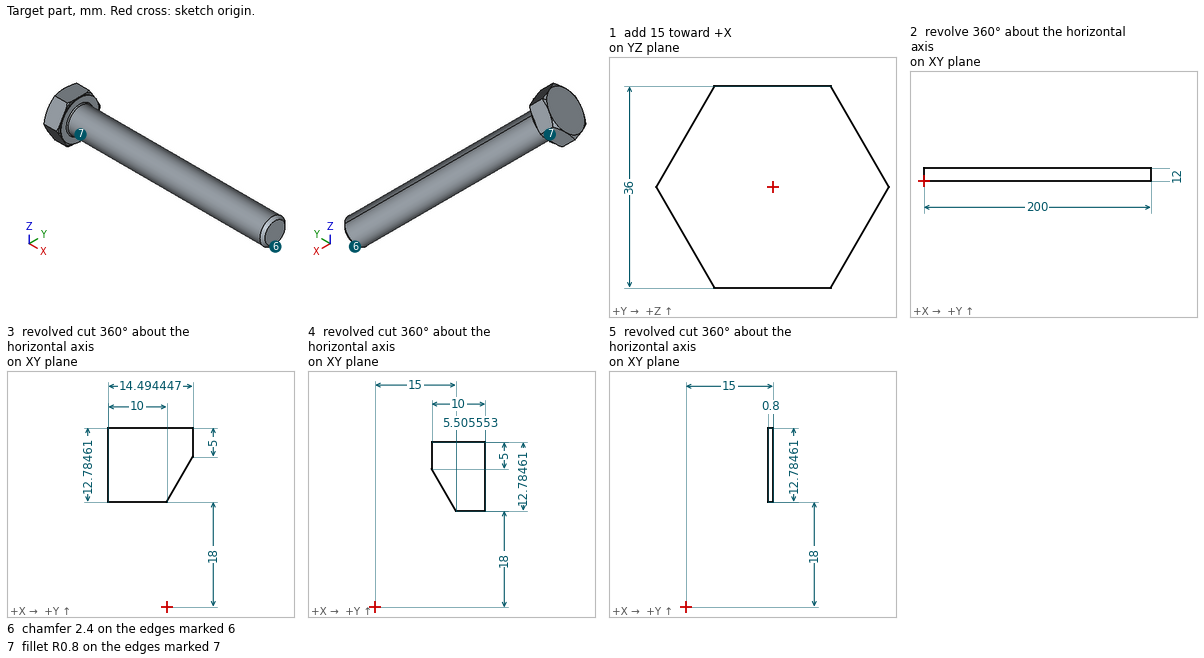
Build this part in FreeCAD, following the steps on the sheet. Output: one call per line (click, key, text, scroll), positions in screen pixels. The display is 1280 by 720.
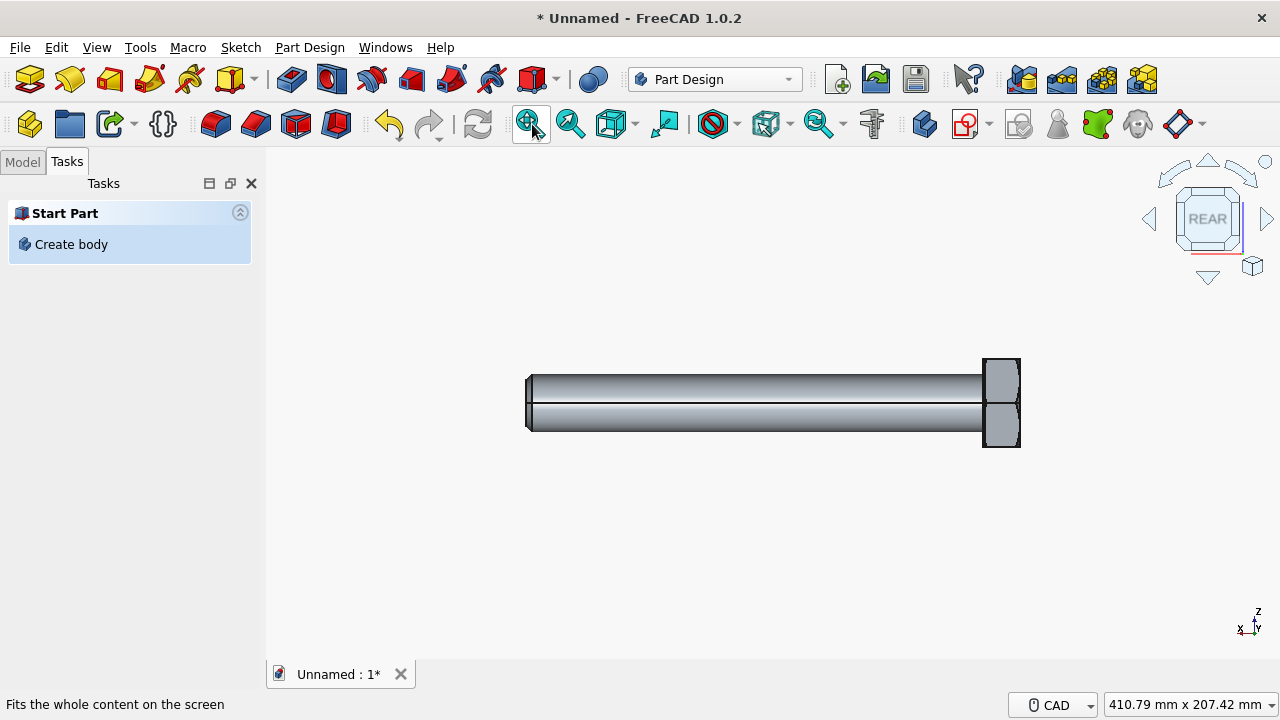
key(6)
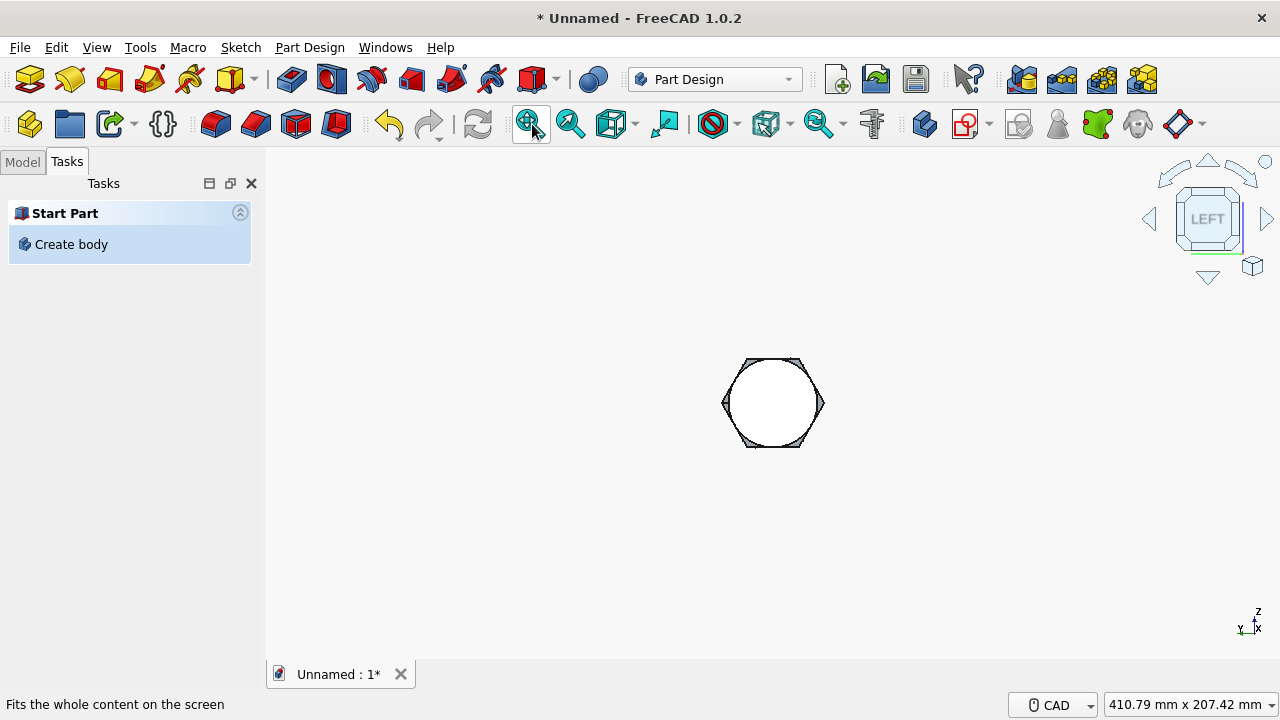
click(532, 124)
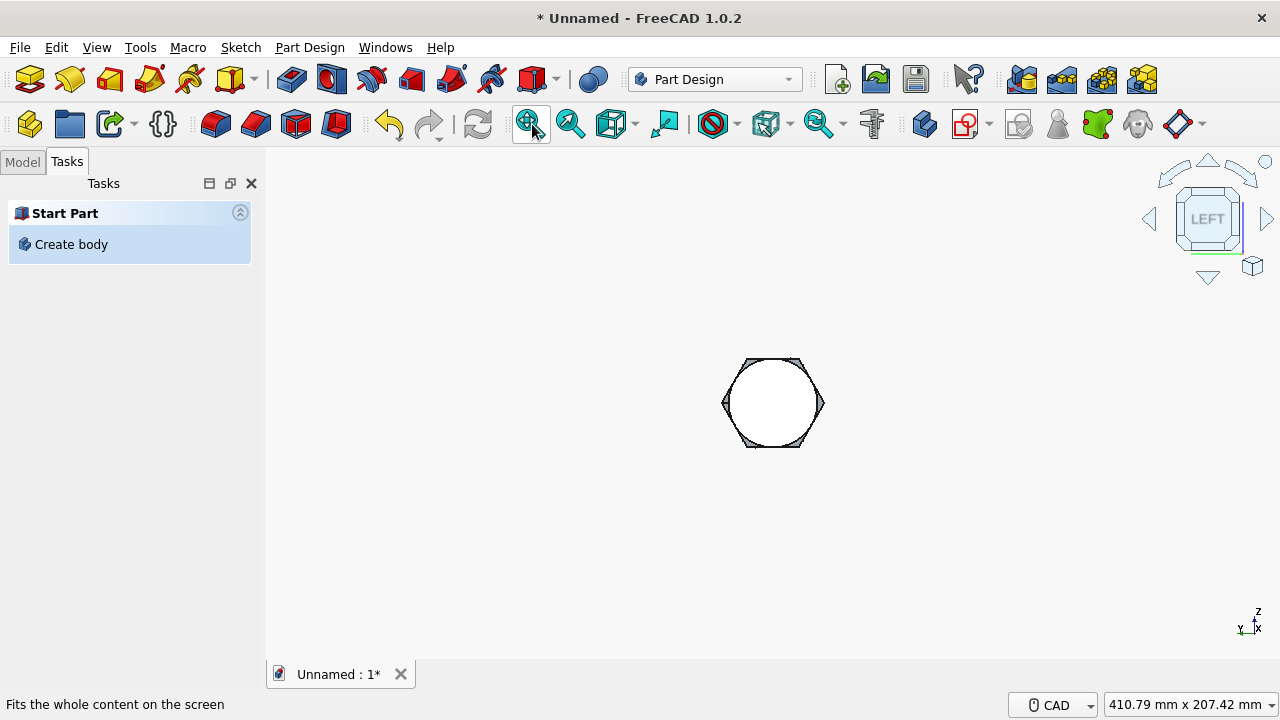
key(v)
key(3)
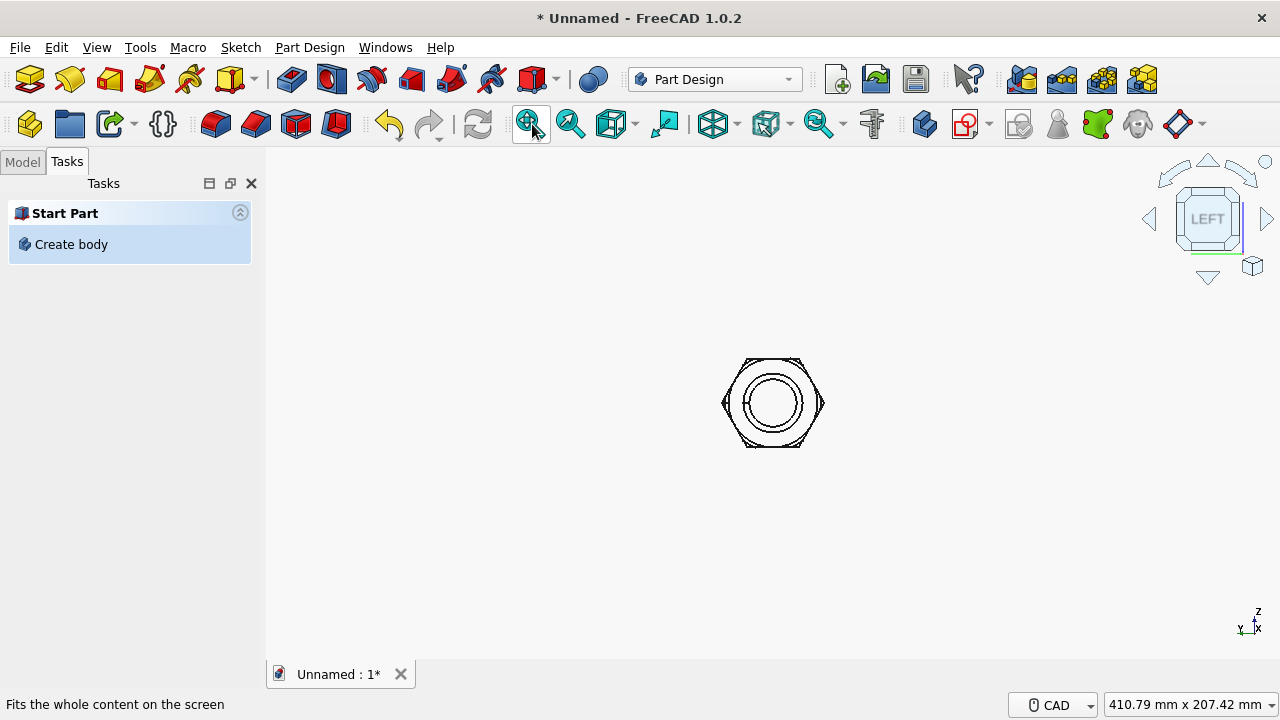
key(0)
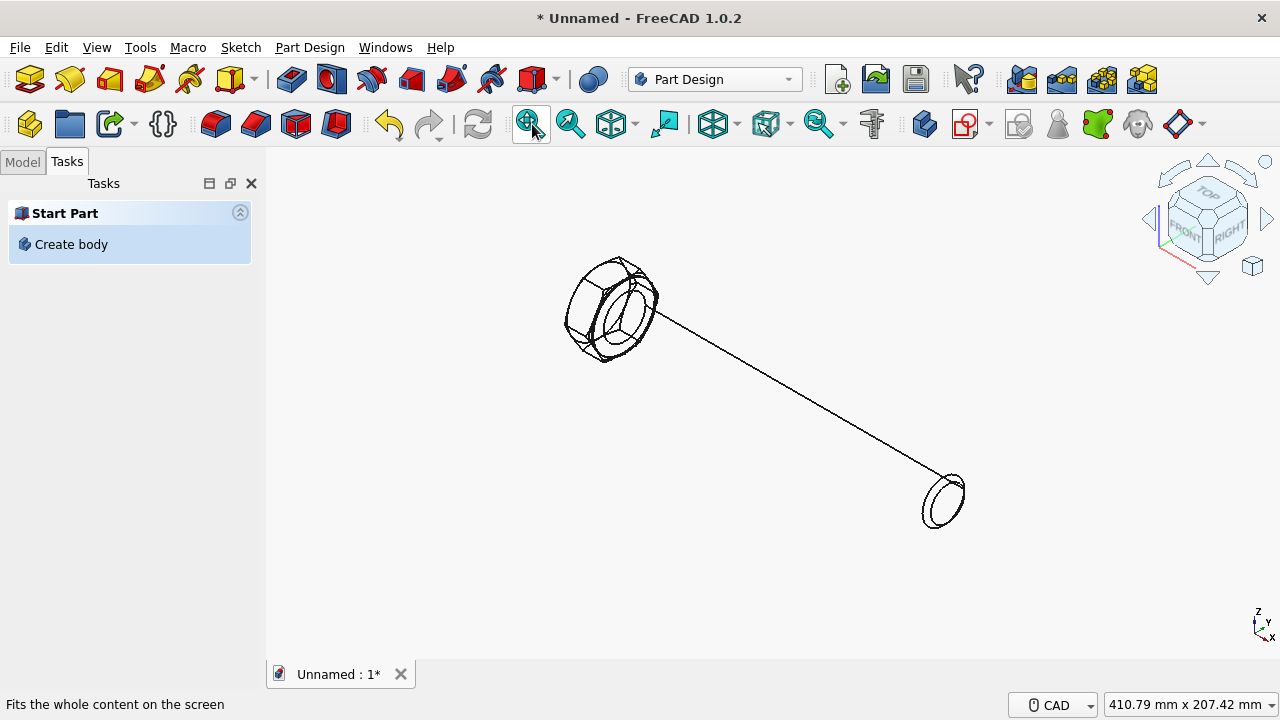
click(604, 328)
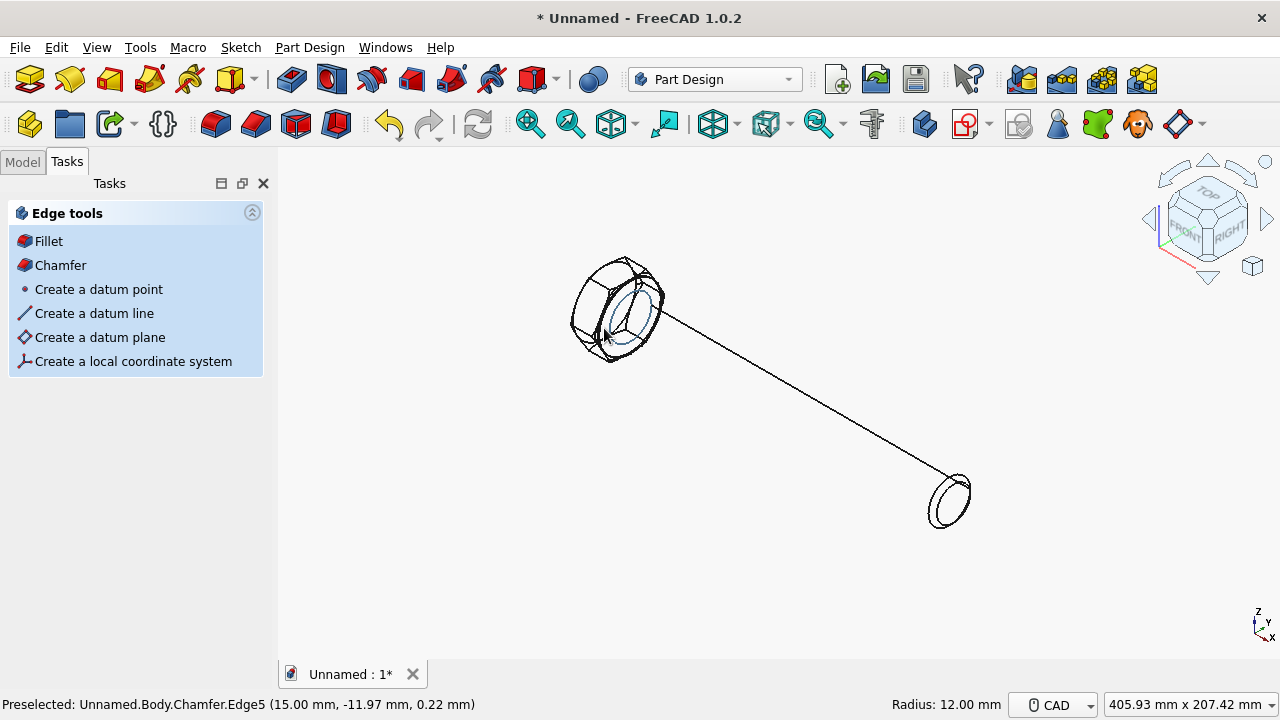
key(v)
key(1)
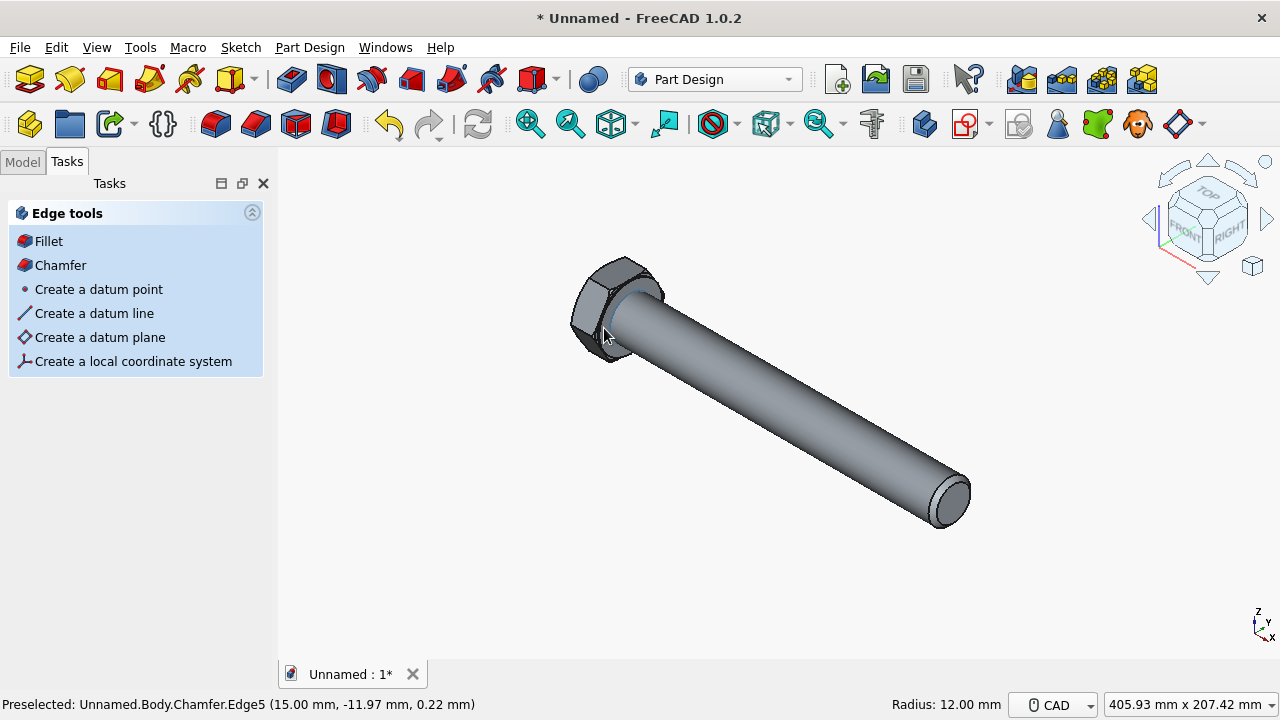
click(216, 124)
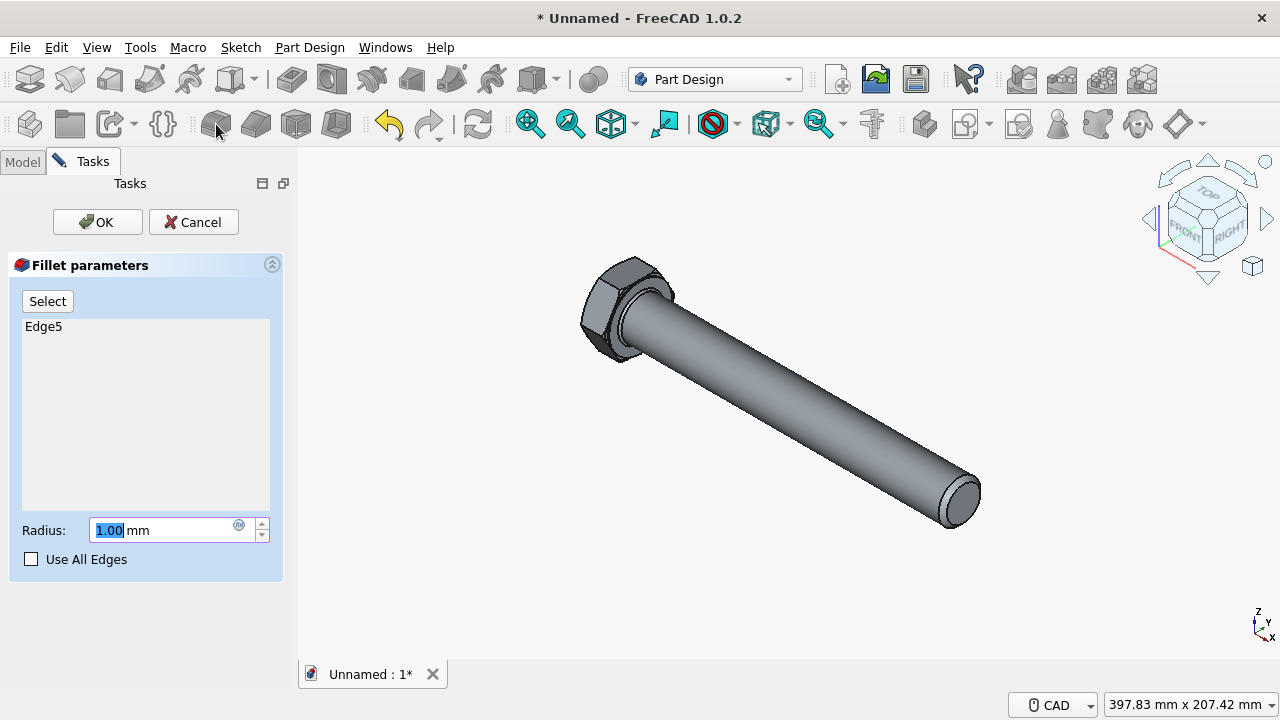
text(0.8)
key(Tab)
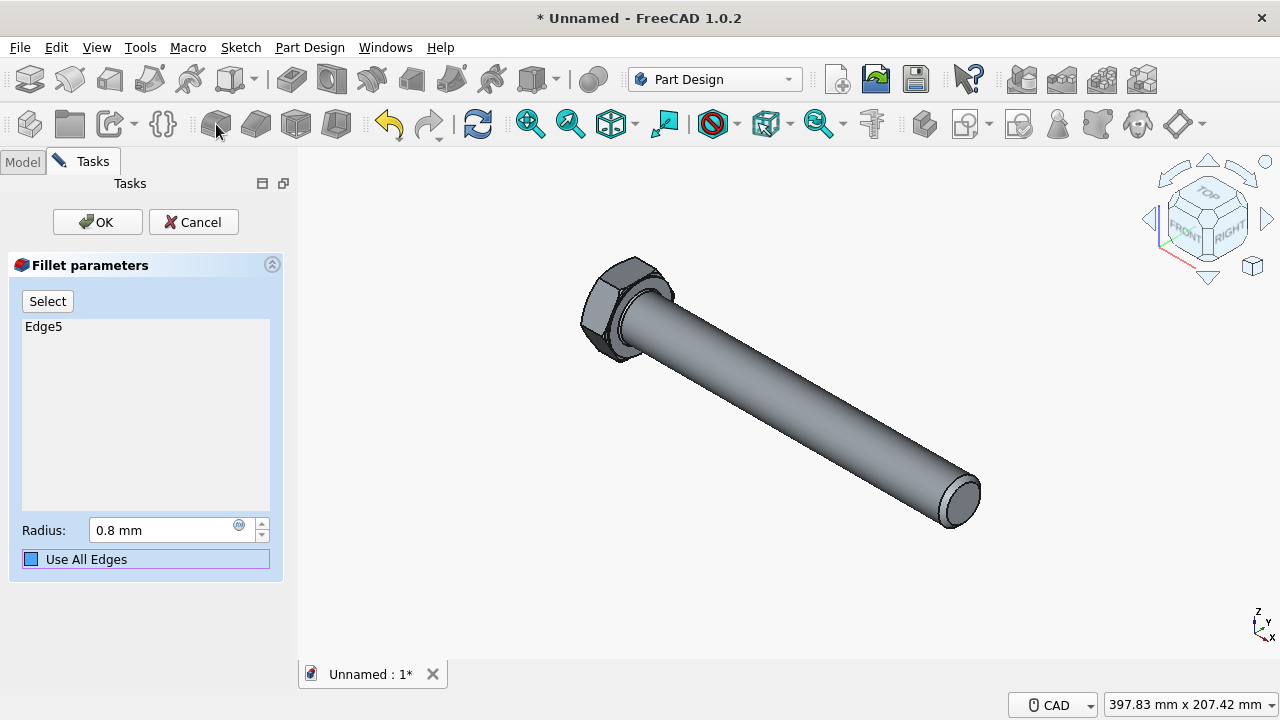
click(98, 222)